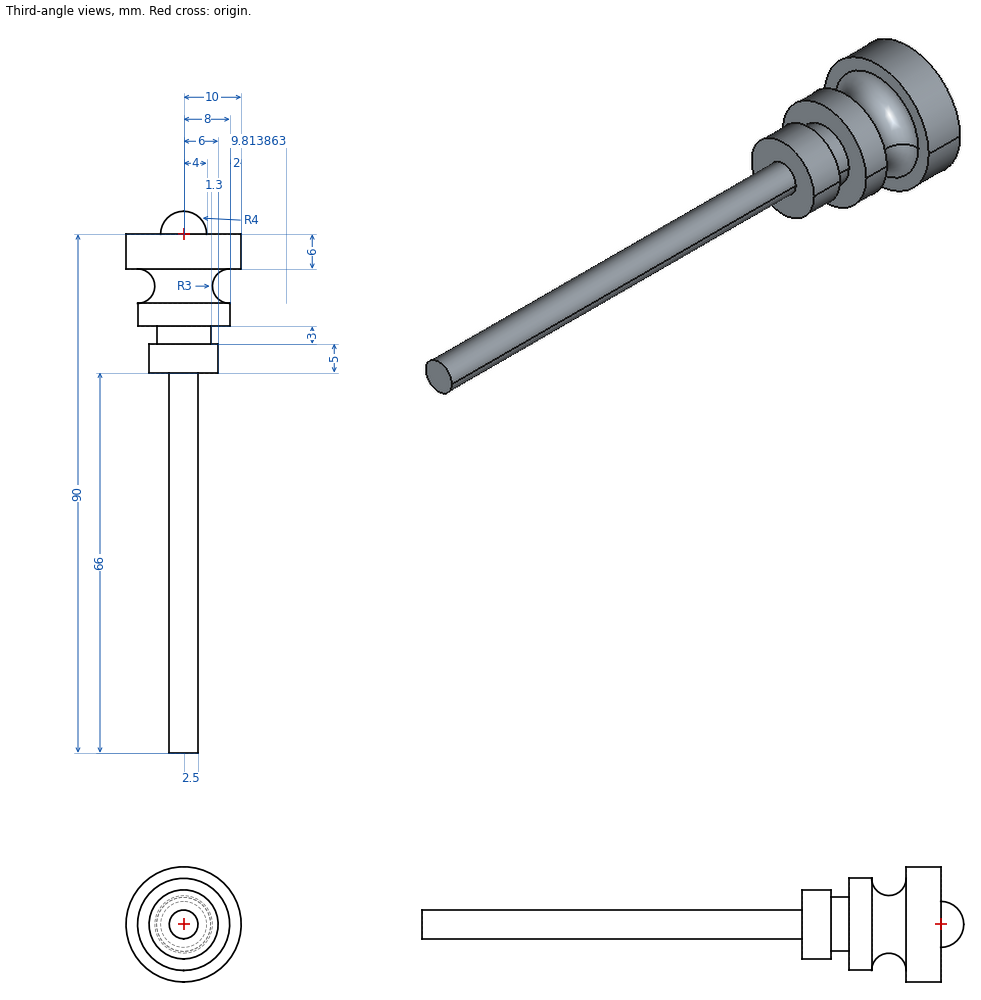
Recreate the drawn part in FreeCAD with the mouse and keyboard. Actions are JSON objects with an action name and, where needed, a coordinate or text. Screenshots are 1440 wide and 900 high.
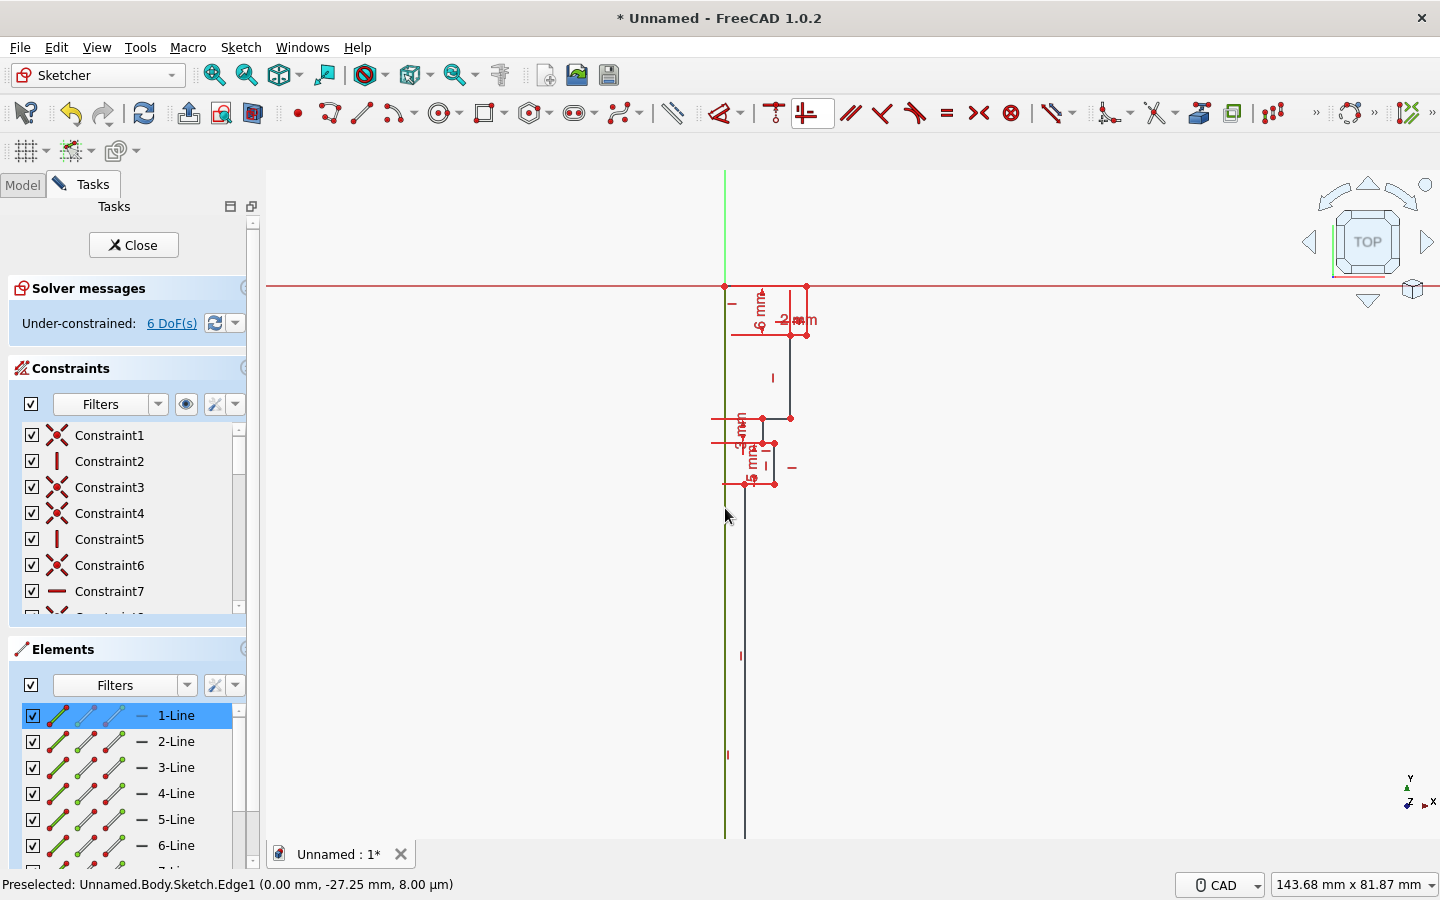
{"action": "key", "text": "i"}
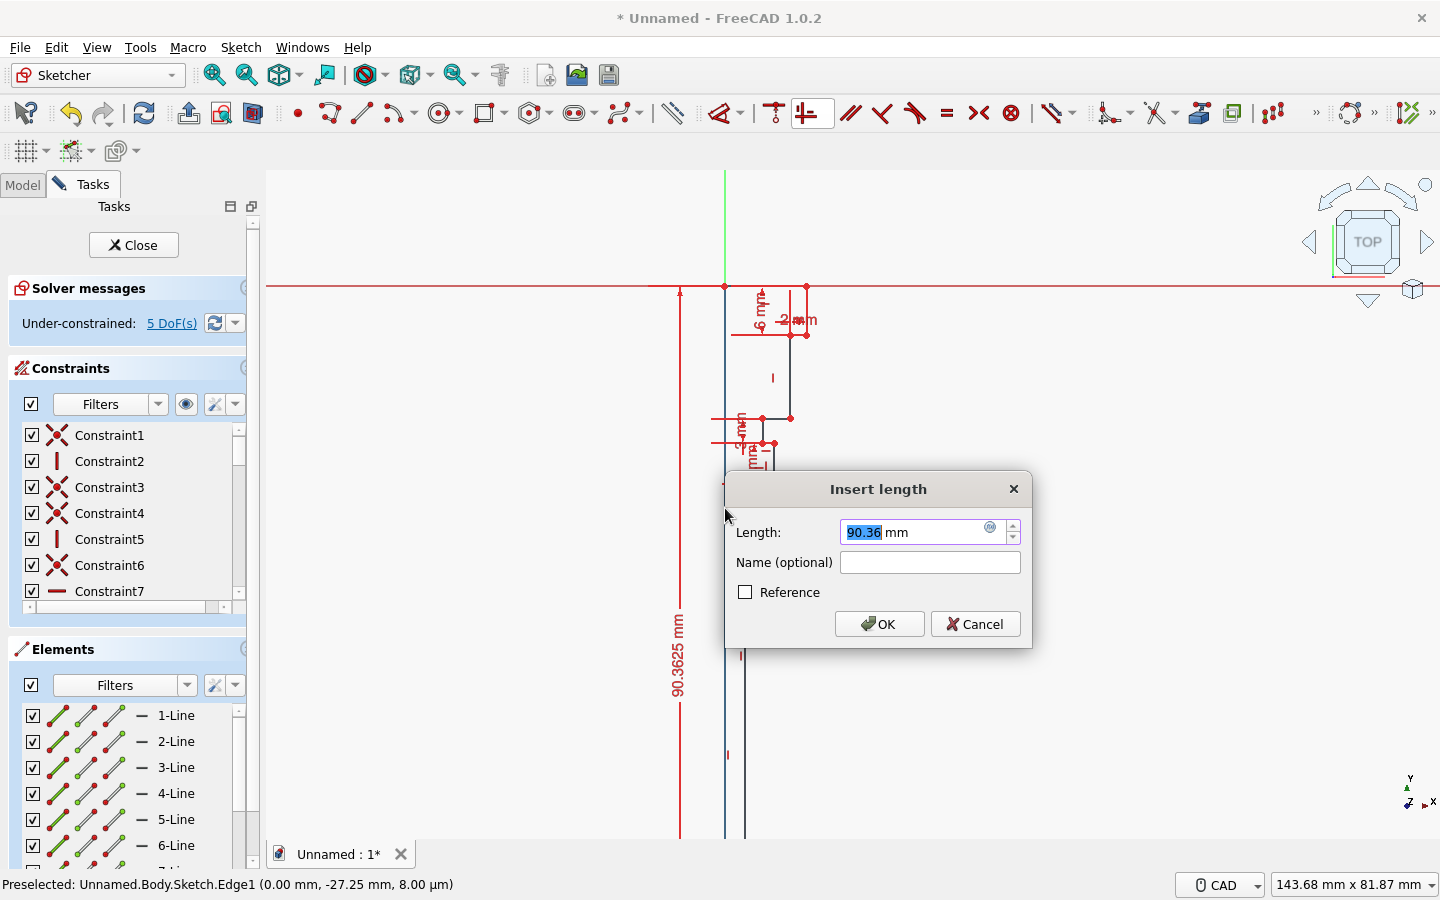
{"action": "type", "text": "90"}
{"action": "key", "text": "Return"}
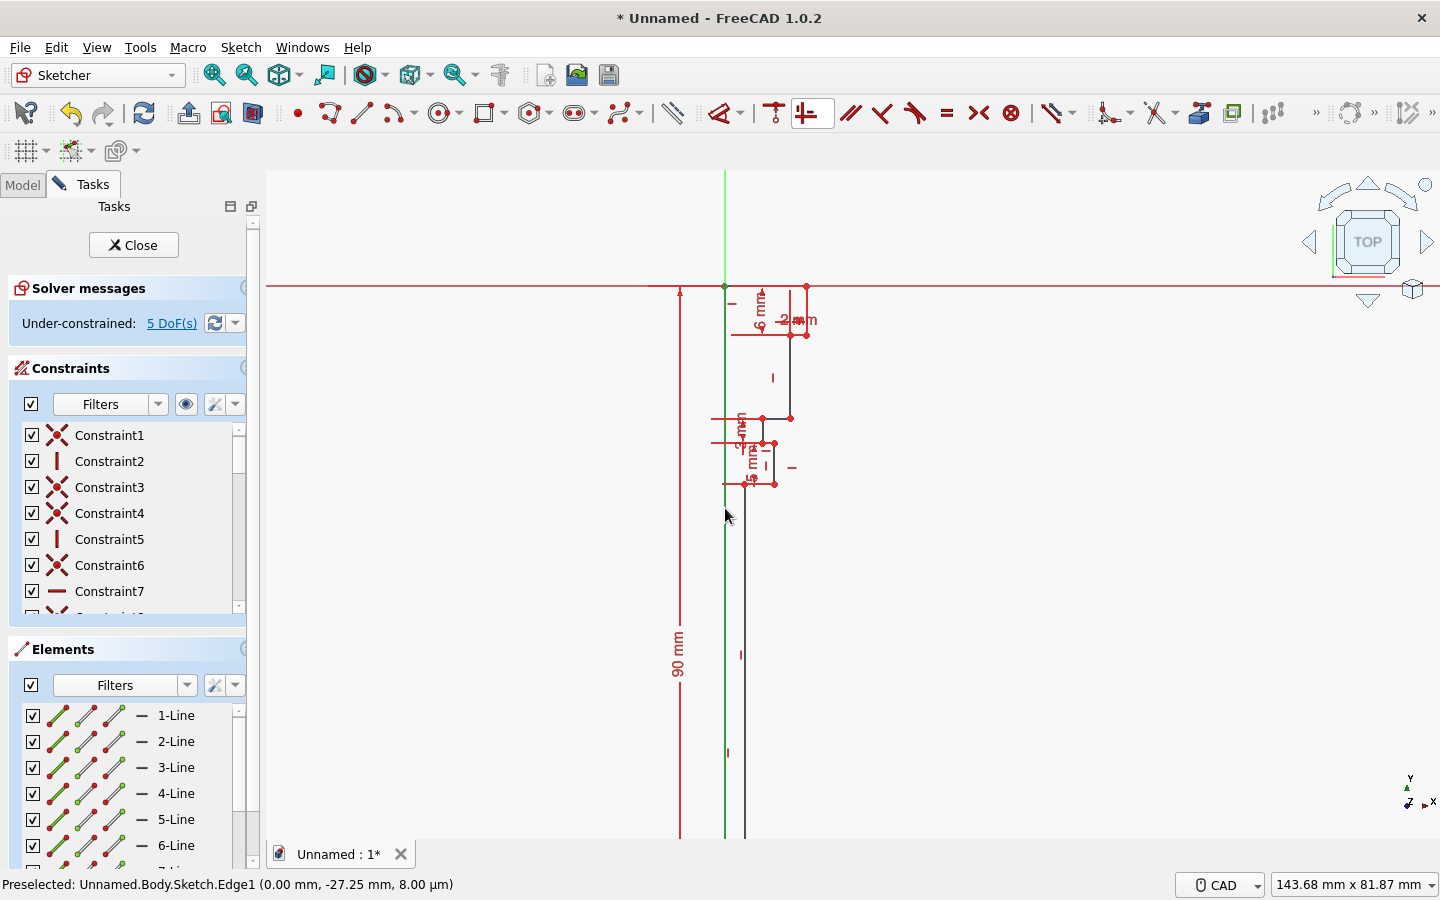
{"action": "left_click", "coordinate": [745, 645]}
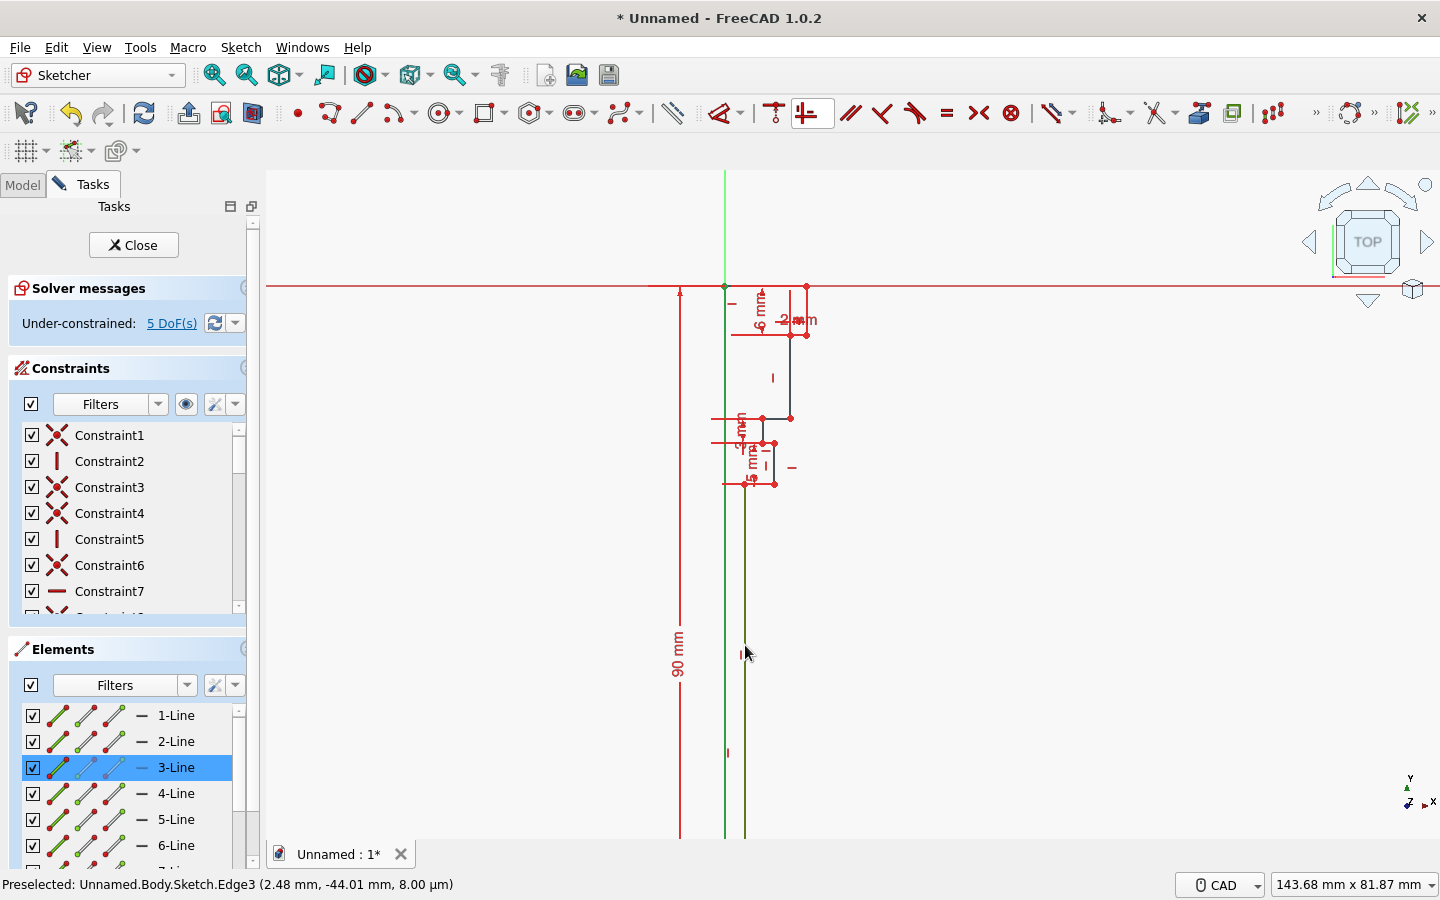
{"action": "left_click", "coordinate": [742, 114]}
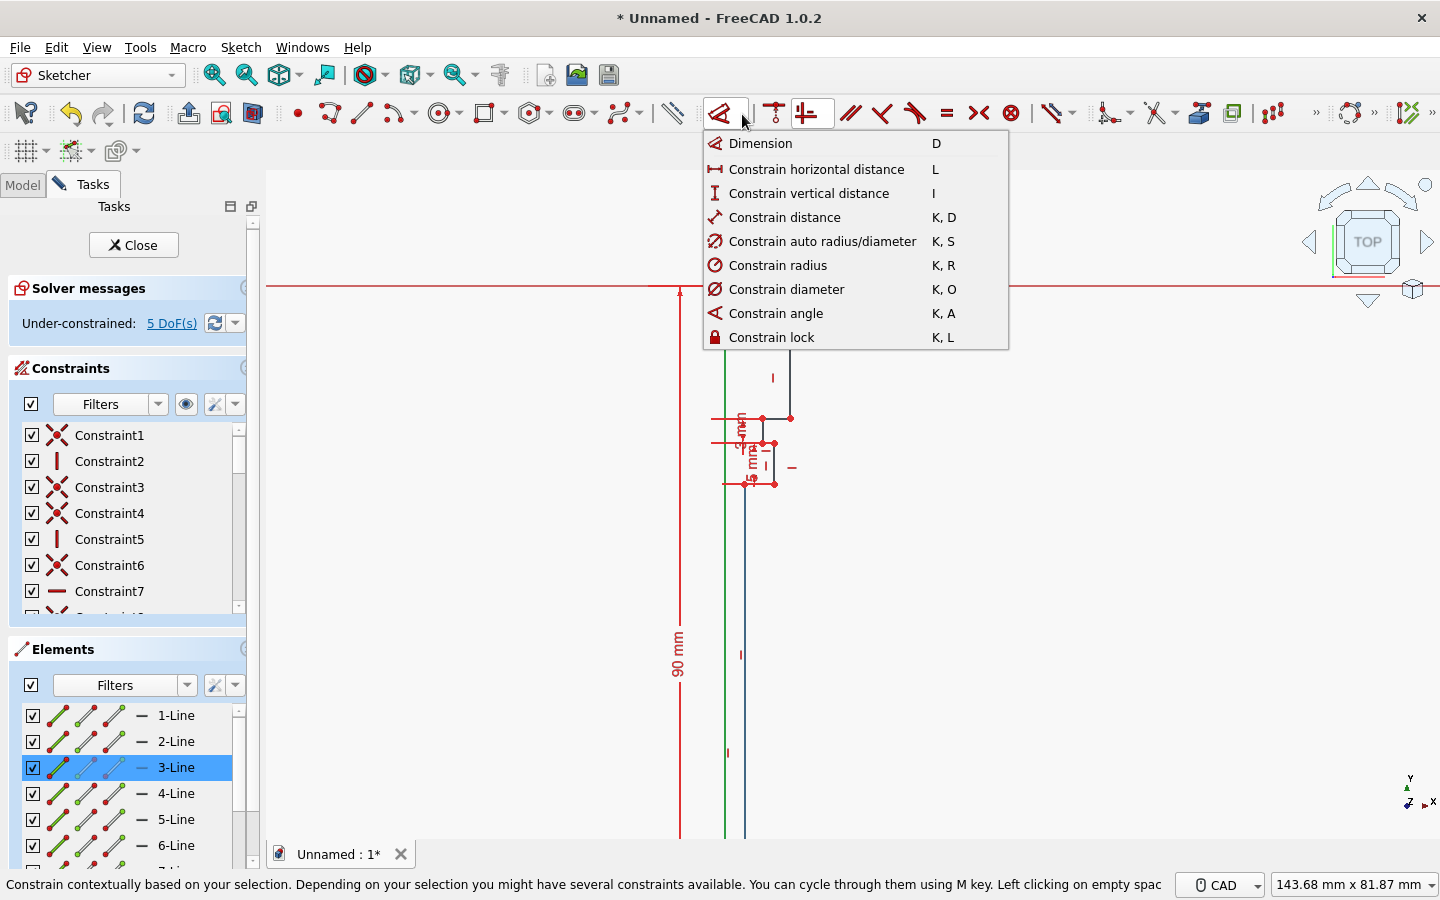
{"action": "left_click", "coordinate": [856, 193]}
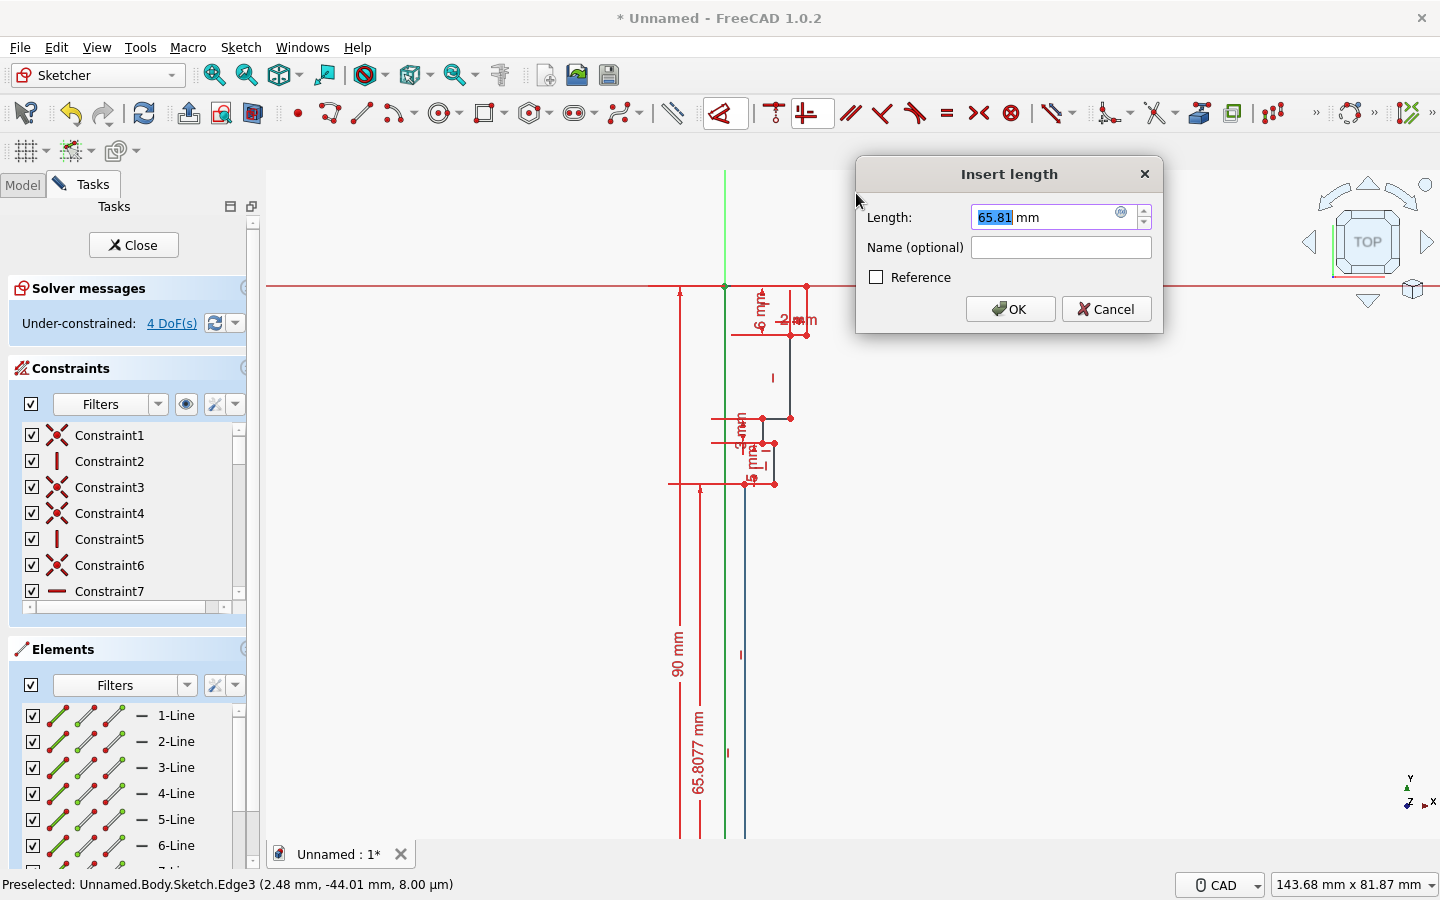
{"action": "type", "text": "66"}
{"action": "key", "text": "Return"}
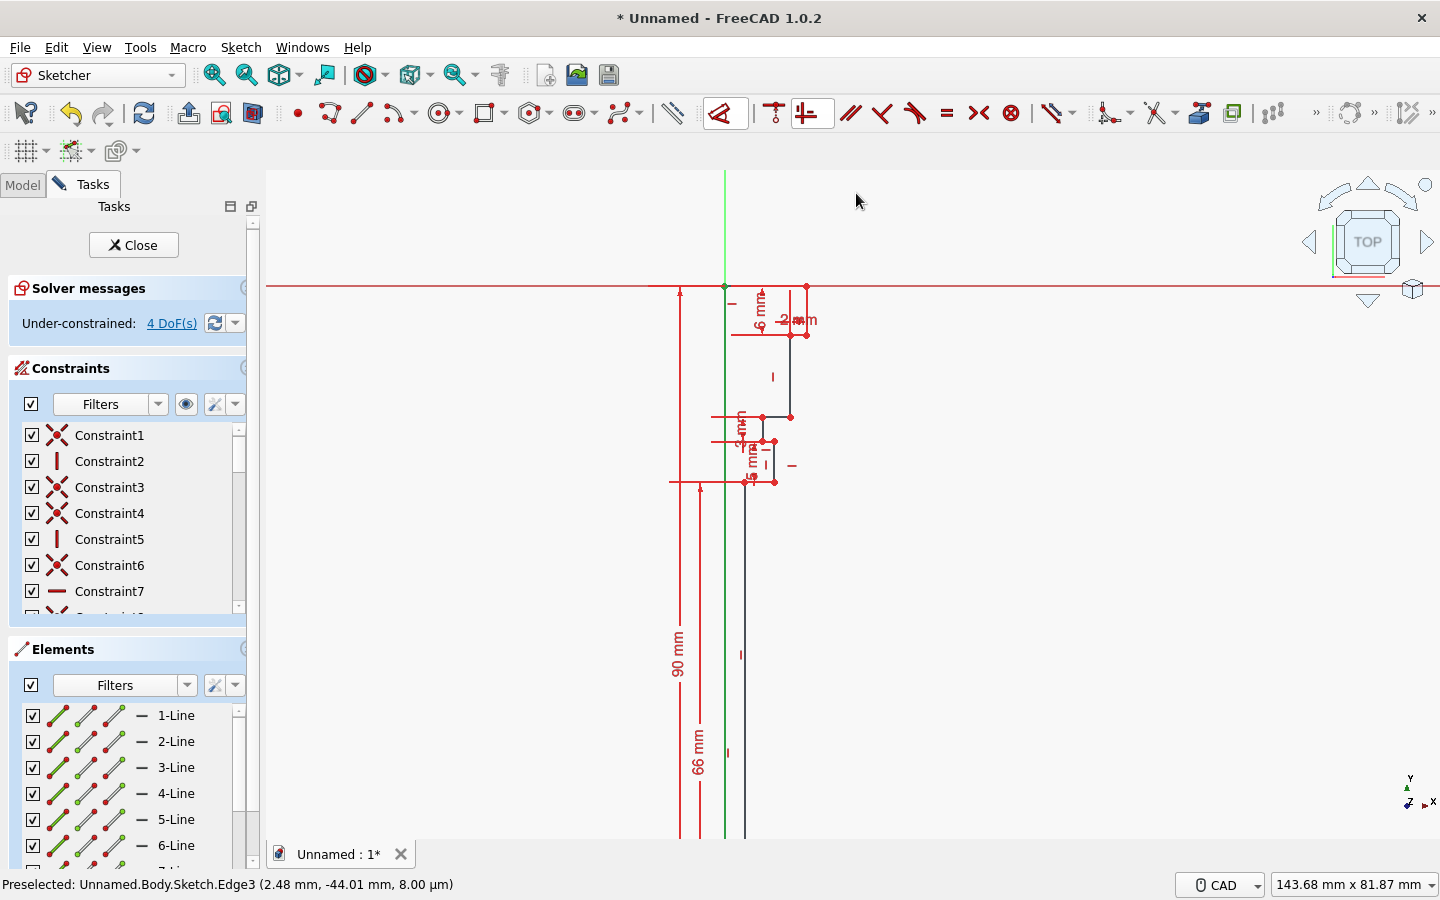
{"action": "left_click", "coordinate": [782, 286]}